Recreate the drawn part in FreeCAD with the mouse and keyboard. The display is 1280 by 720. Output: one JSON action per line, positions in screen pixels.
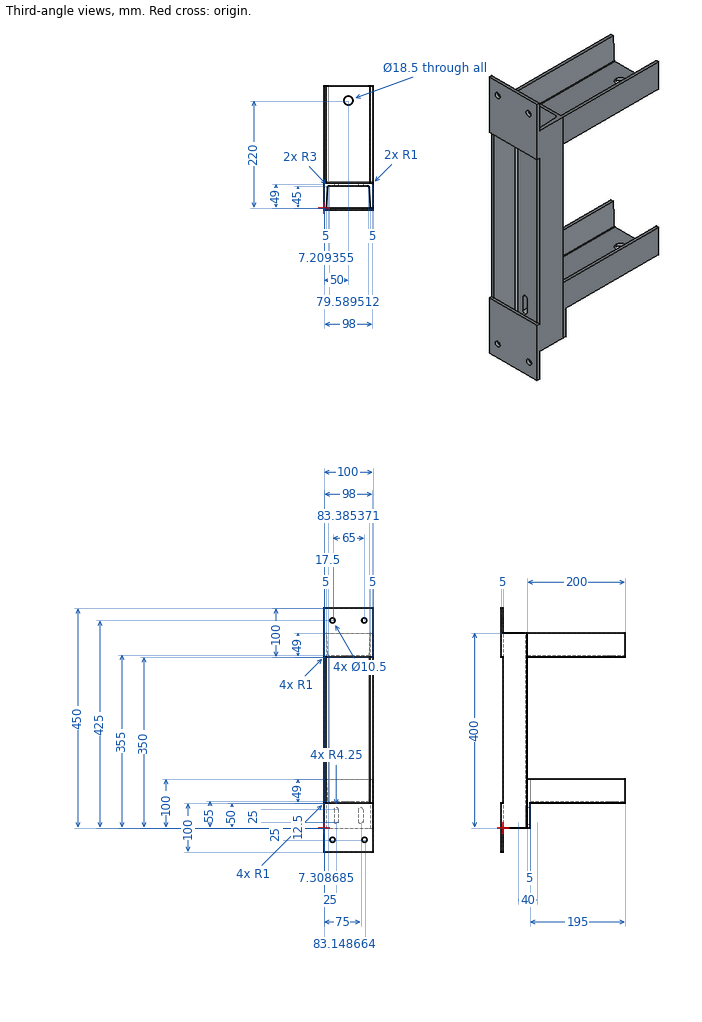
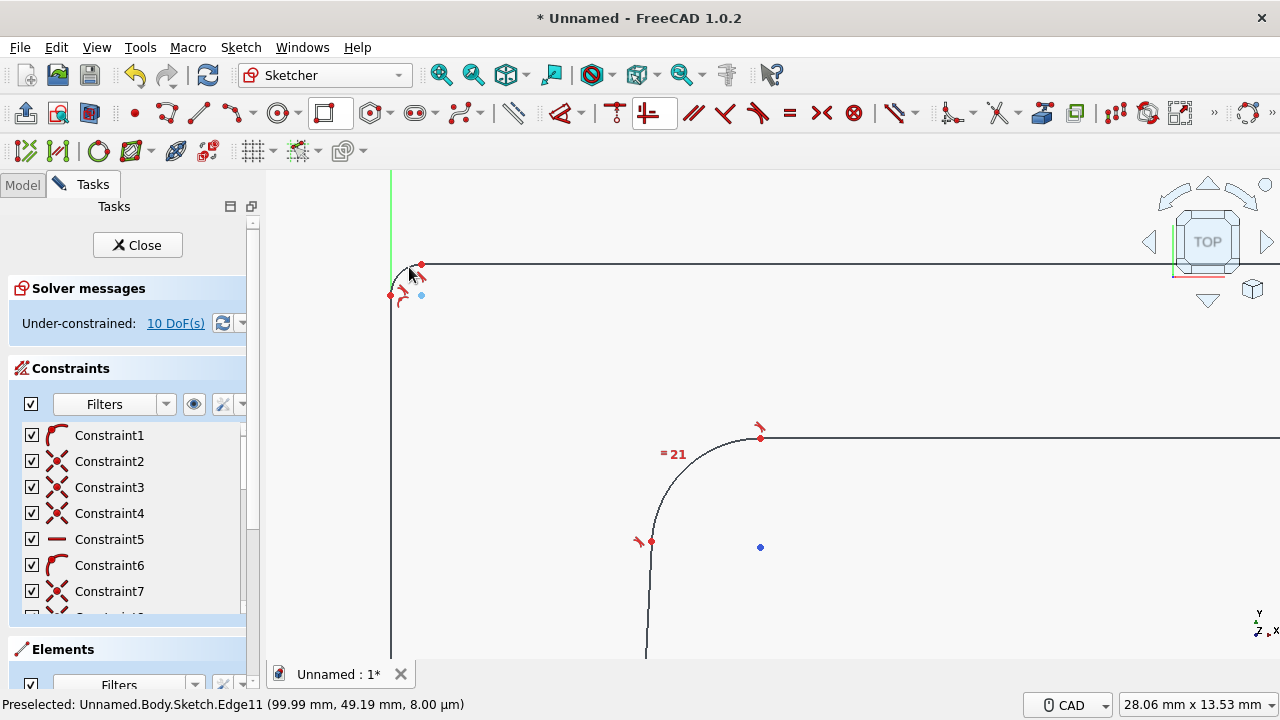
{"action": "left_click", "coordinate": [408, 268]}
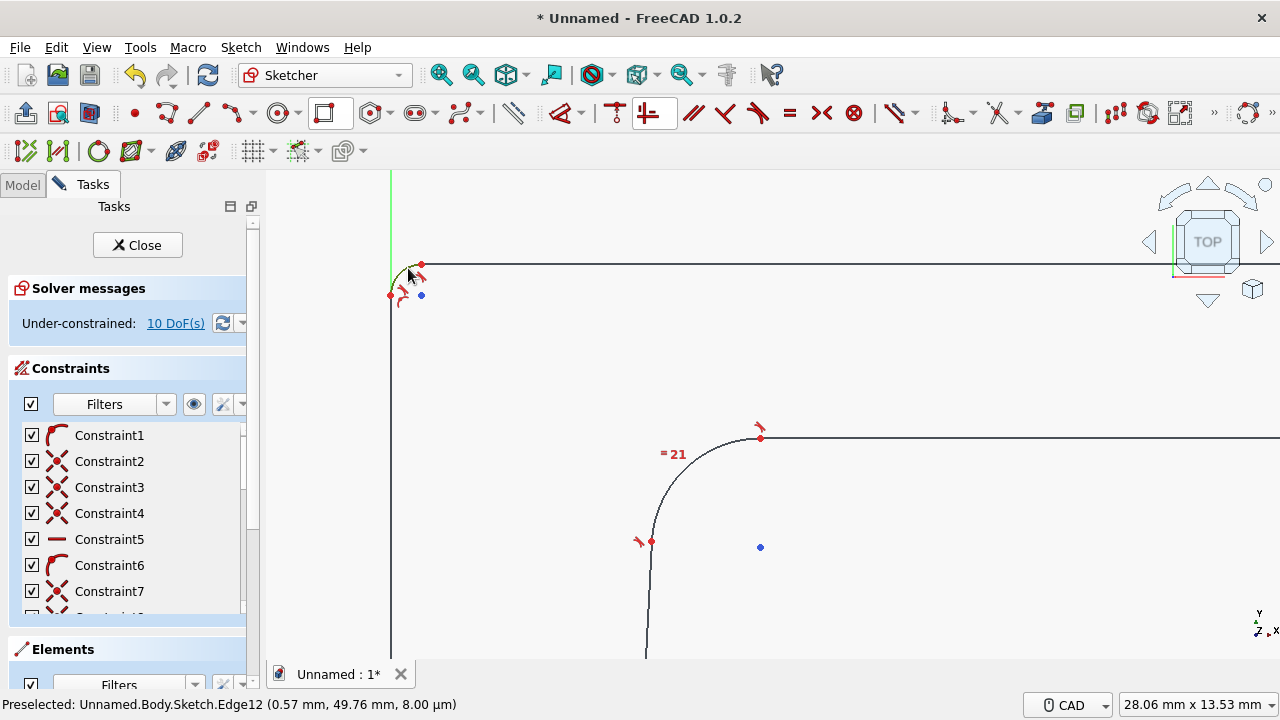
{"action": "left_click", "coordinate": [790, 114]}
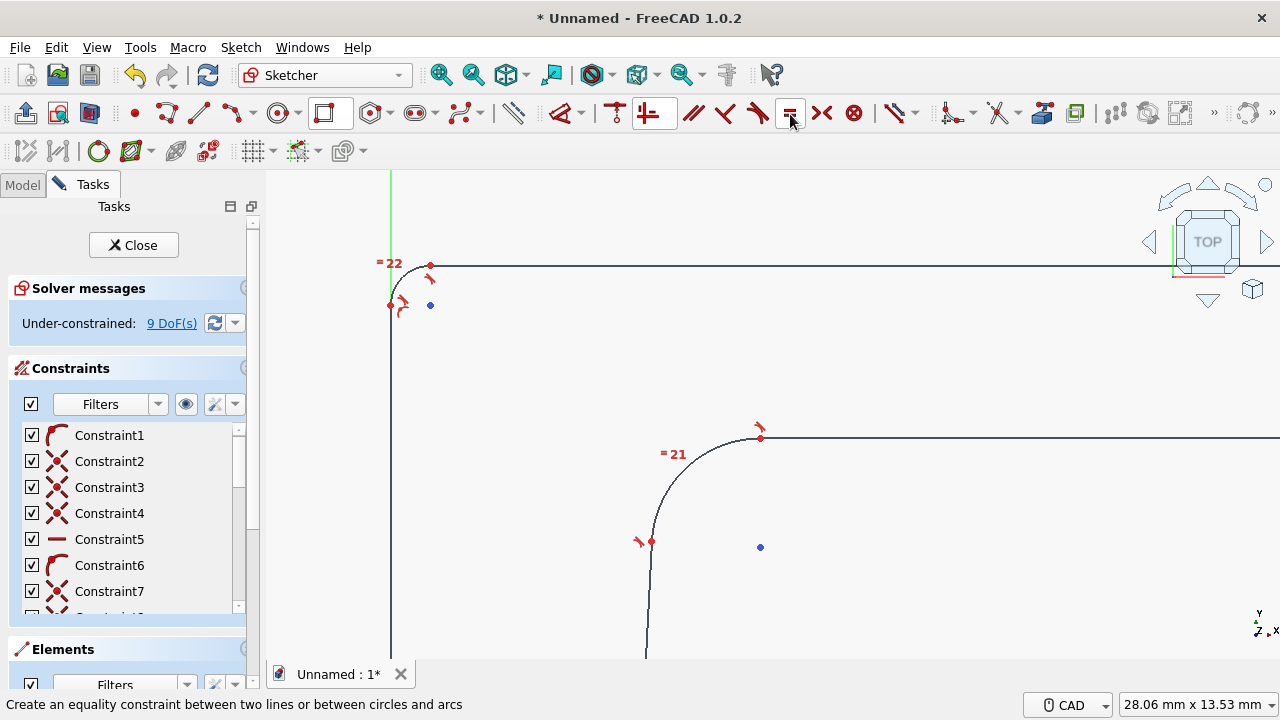
{"action": "left_click", "coordinate": [713, 450]}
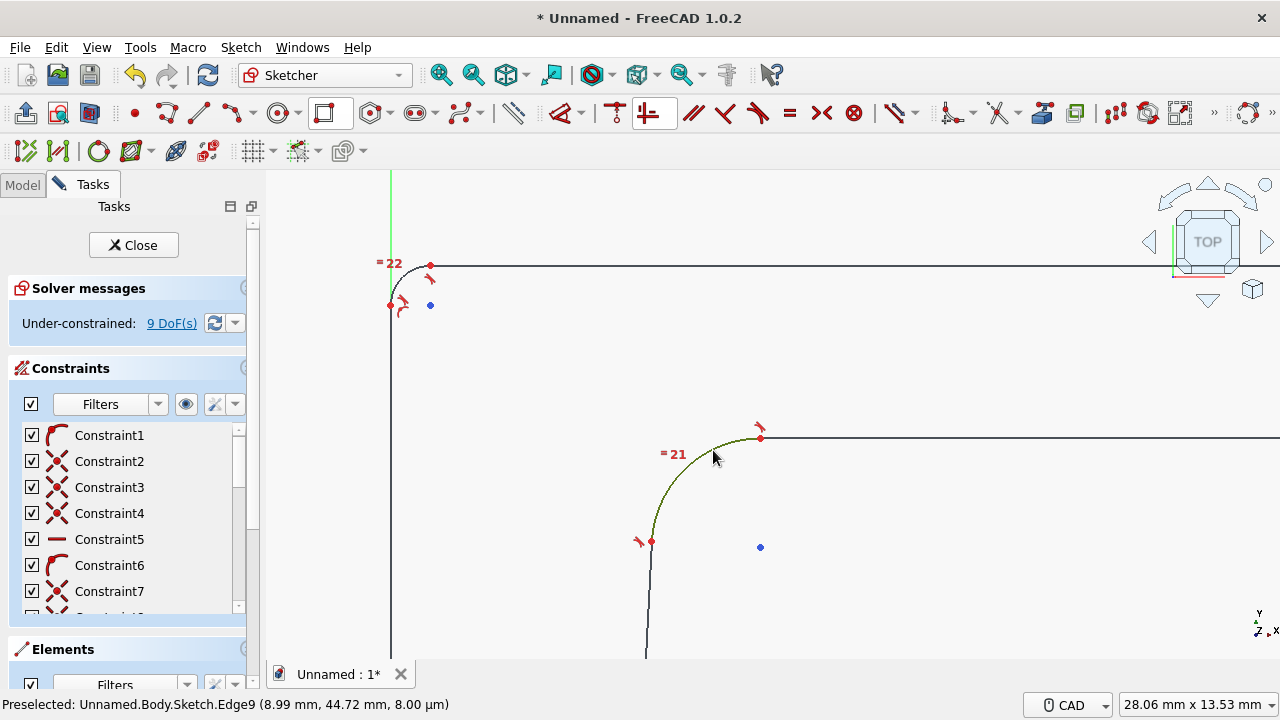
{"action": "left_click", "coordinate": [584, 114]}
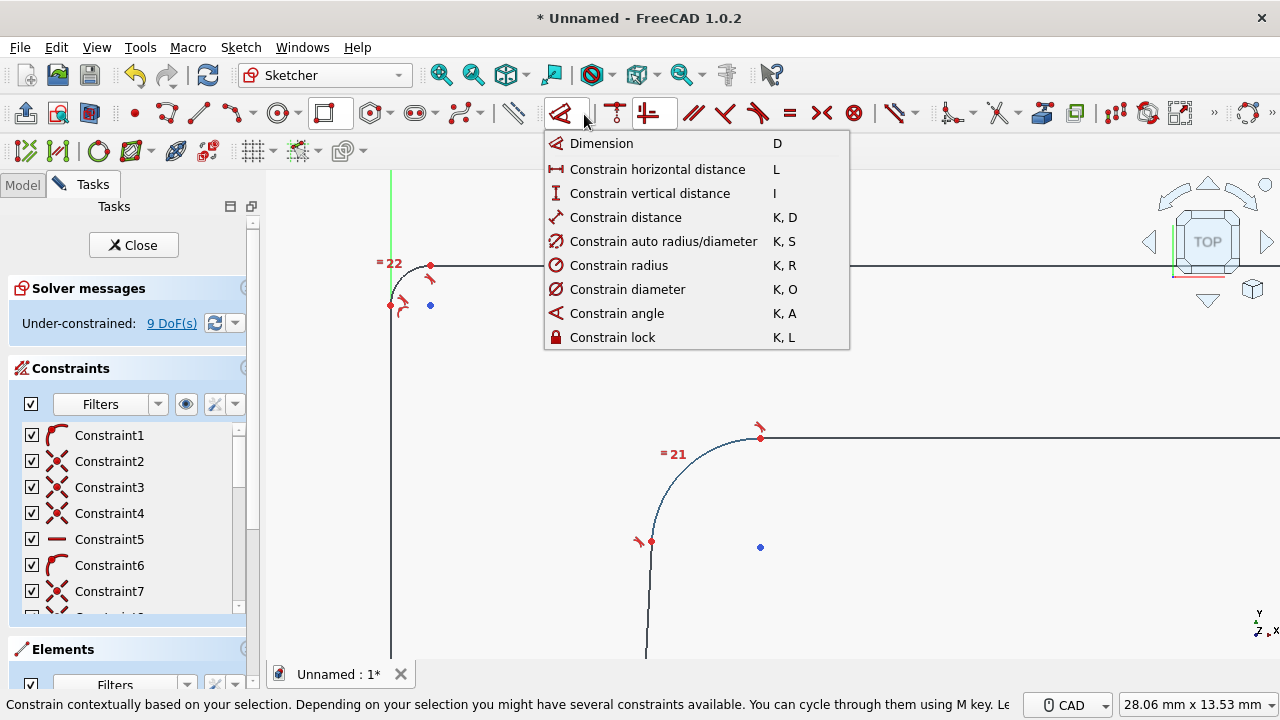
{"action": "left_click", "coordinate": [697, 265]}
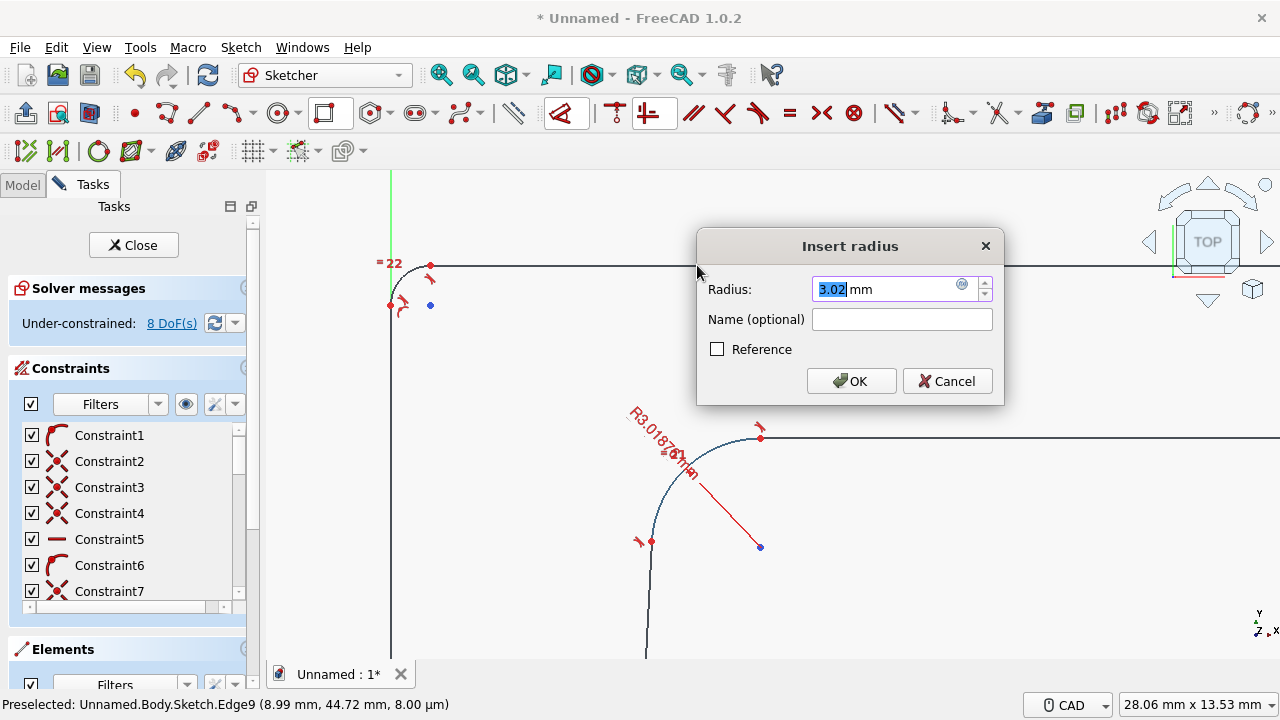
{"action": "type", "text": "3"}
{"action": "key", "text": "Return"}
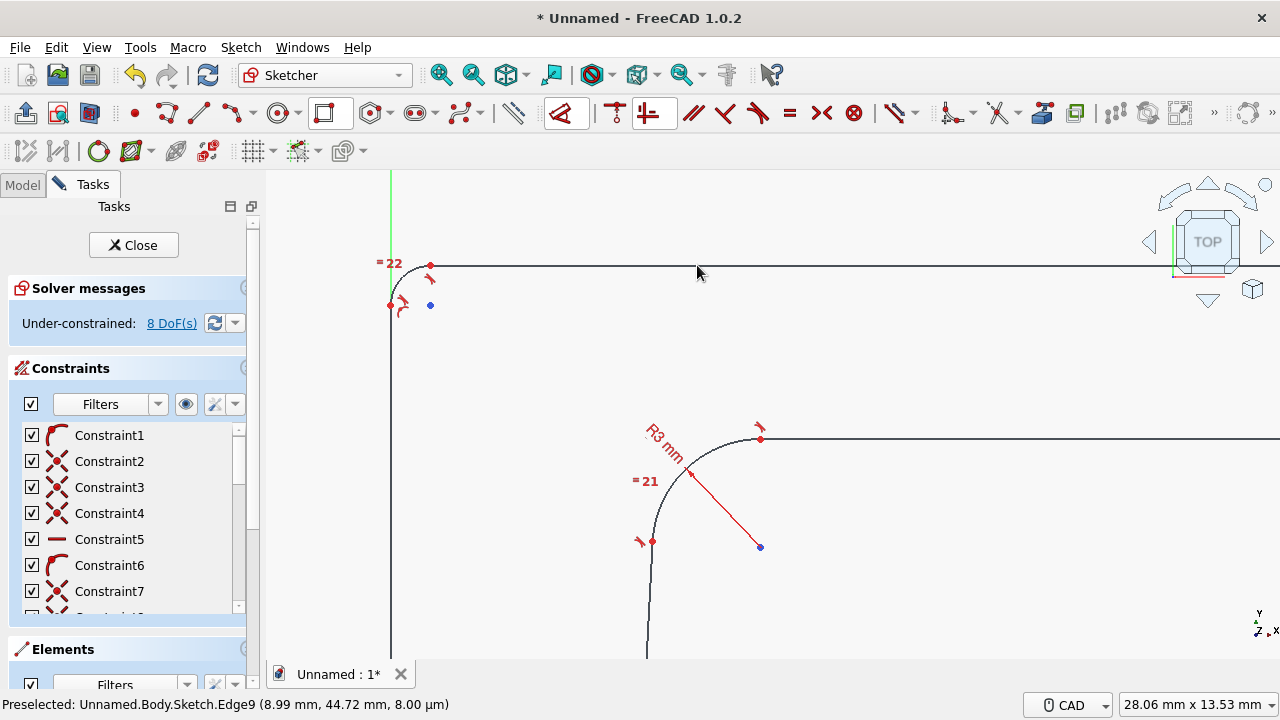
{"action": "scroll", "coordinate": [409, 267], "scroll_direction": "down", "scroll_amount": 9}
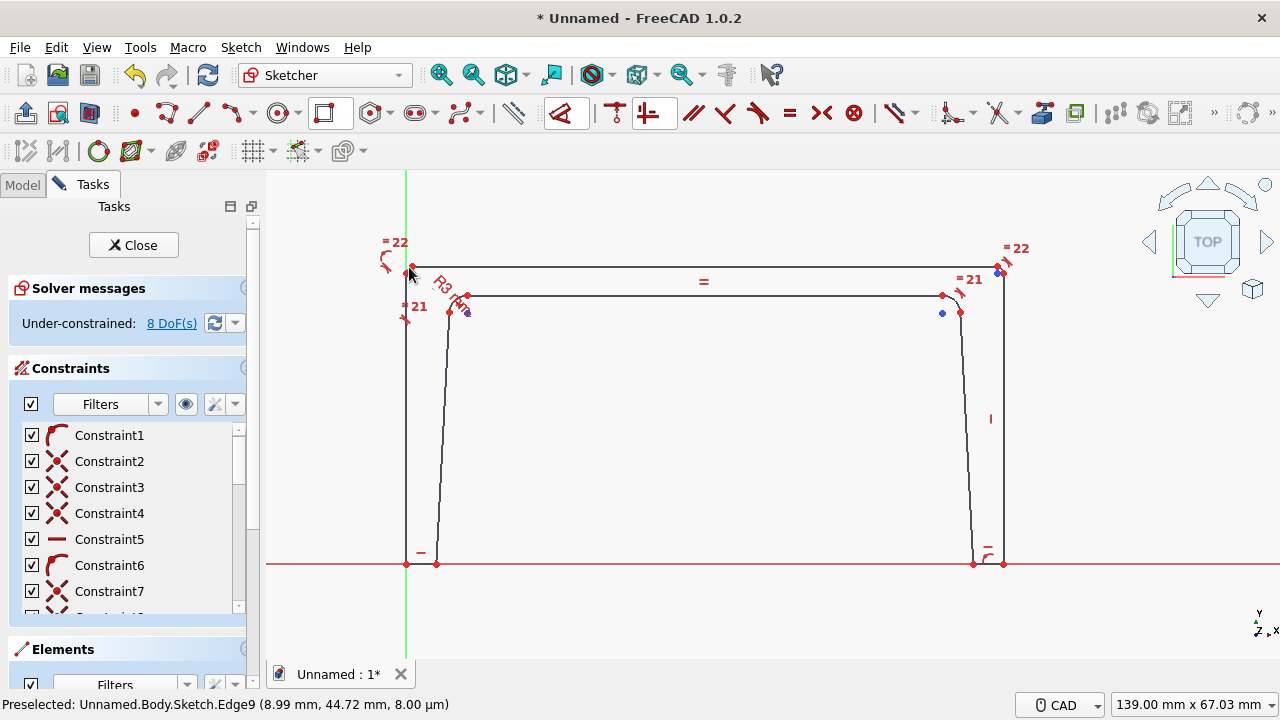
{"action": "scroll", "coordinate": [1003, 271], "scroll_direction": "up", "scroll_amount": 10}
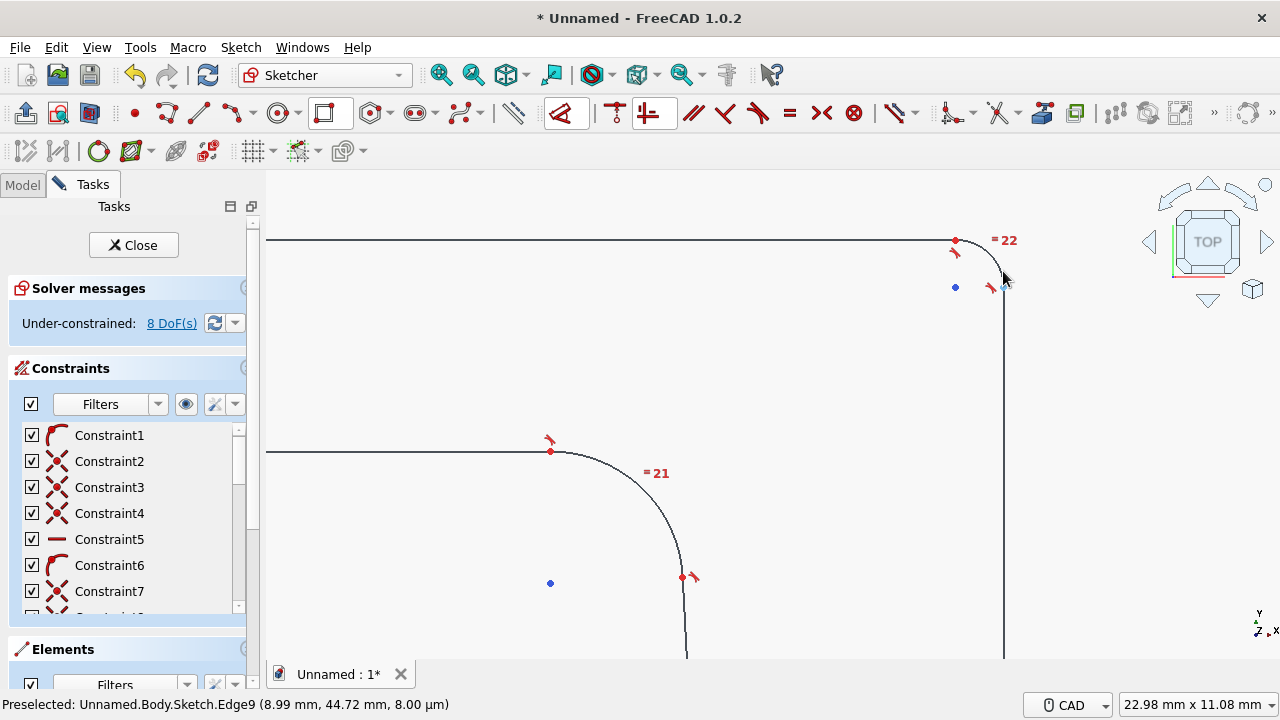
{"action": "left_click", "coordinate": [999, 266]}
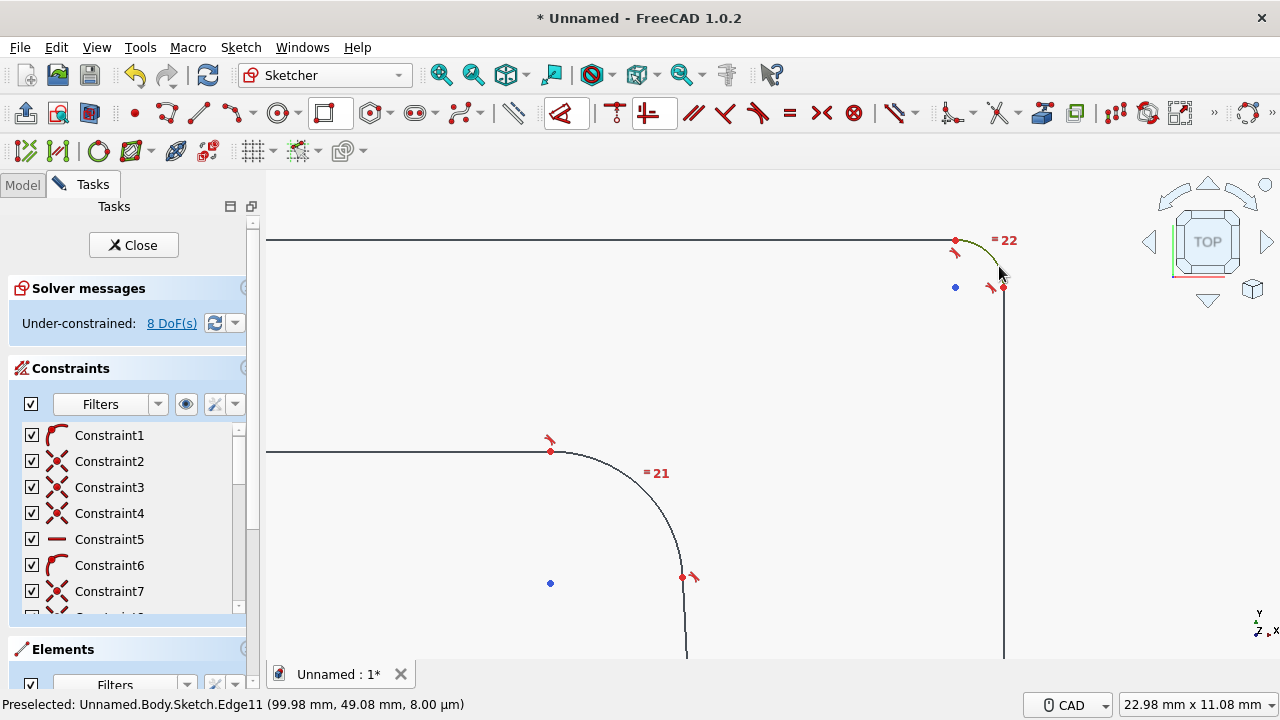
{"action": "left_click", "coordinate": [584, 114]}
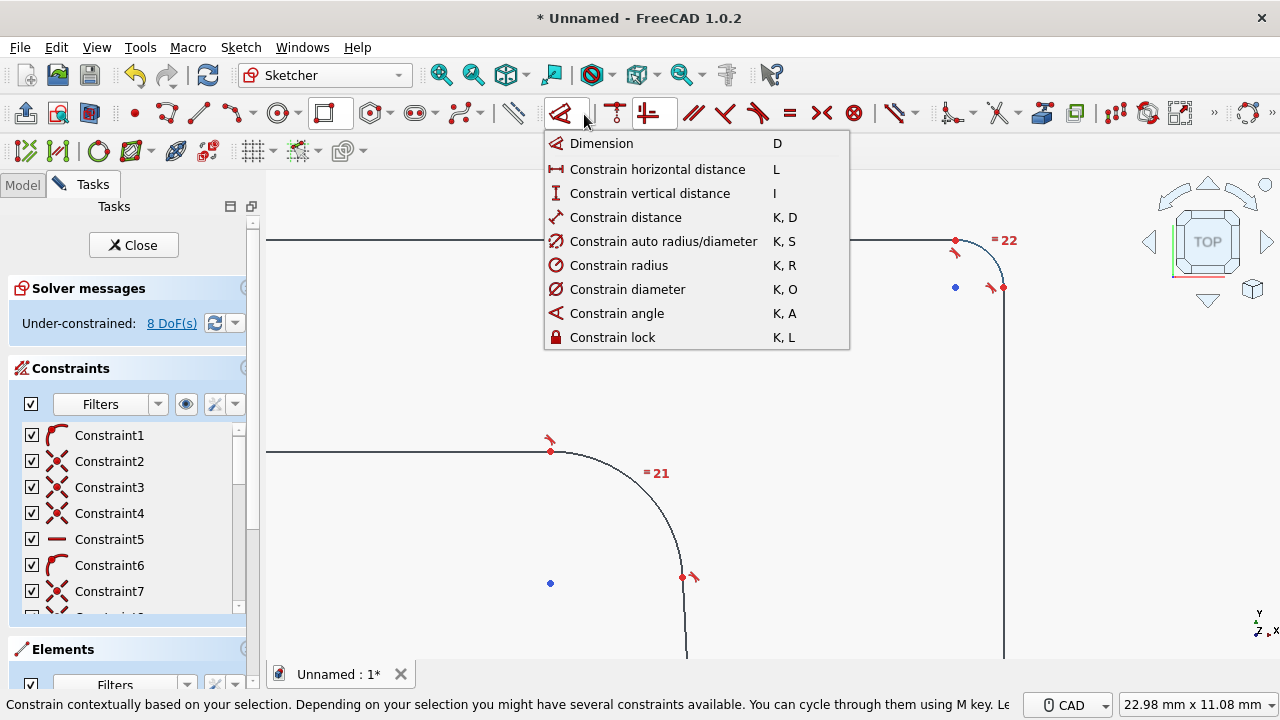
{"action": "left_click", "coordinate": [697, 265]}